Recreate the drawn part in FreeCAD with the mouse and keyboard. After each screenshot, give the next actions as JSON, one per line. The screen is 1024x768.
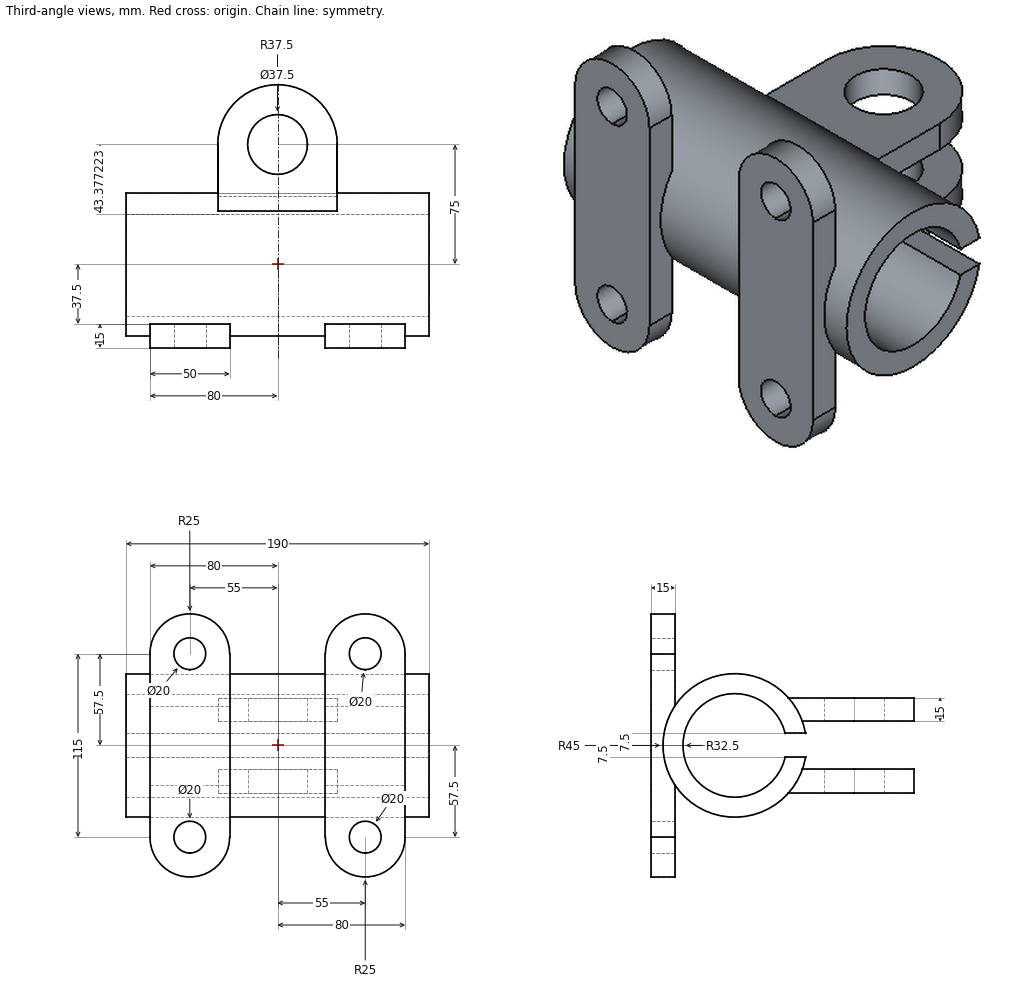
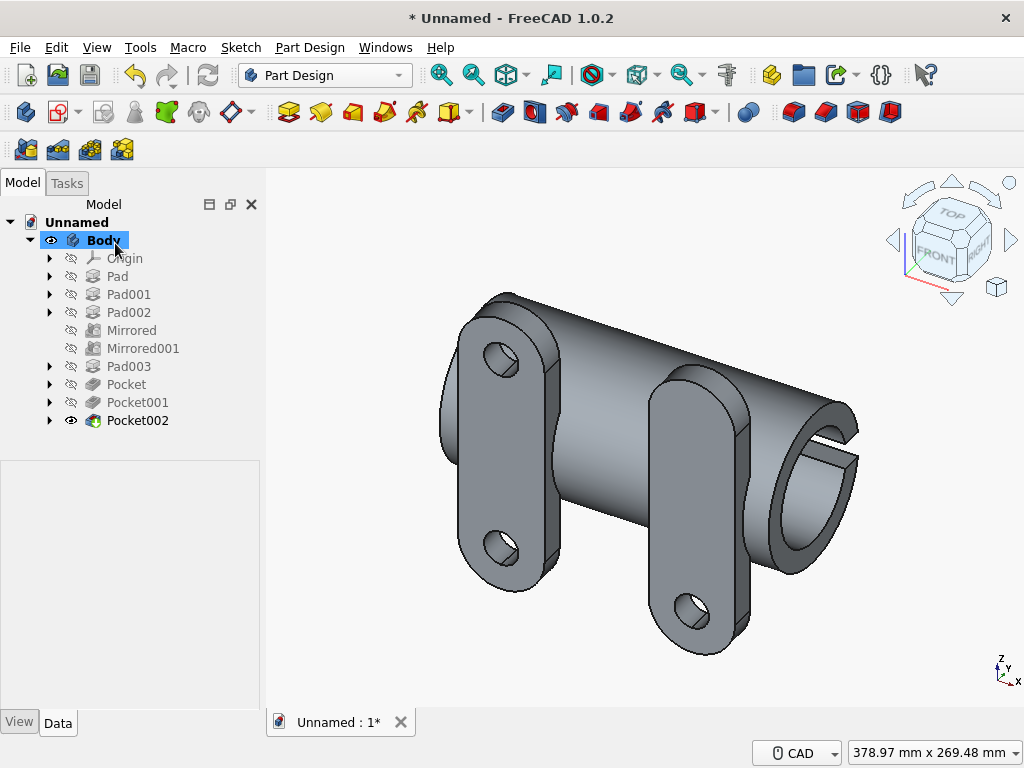
{"action": "left_click", "coordinate": [692, 516]}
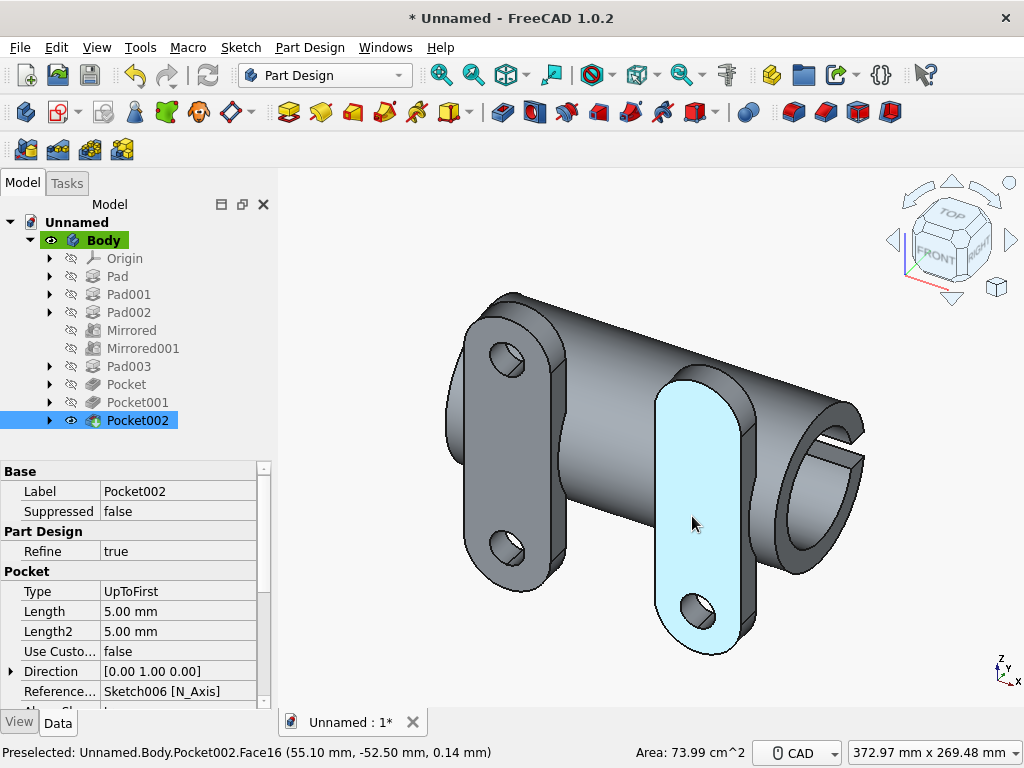
{"action": "left_click", "coordinate": [58, 112]}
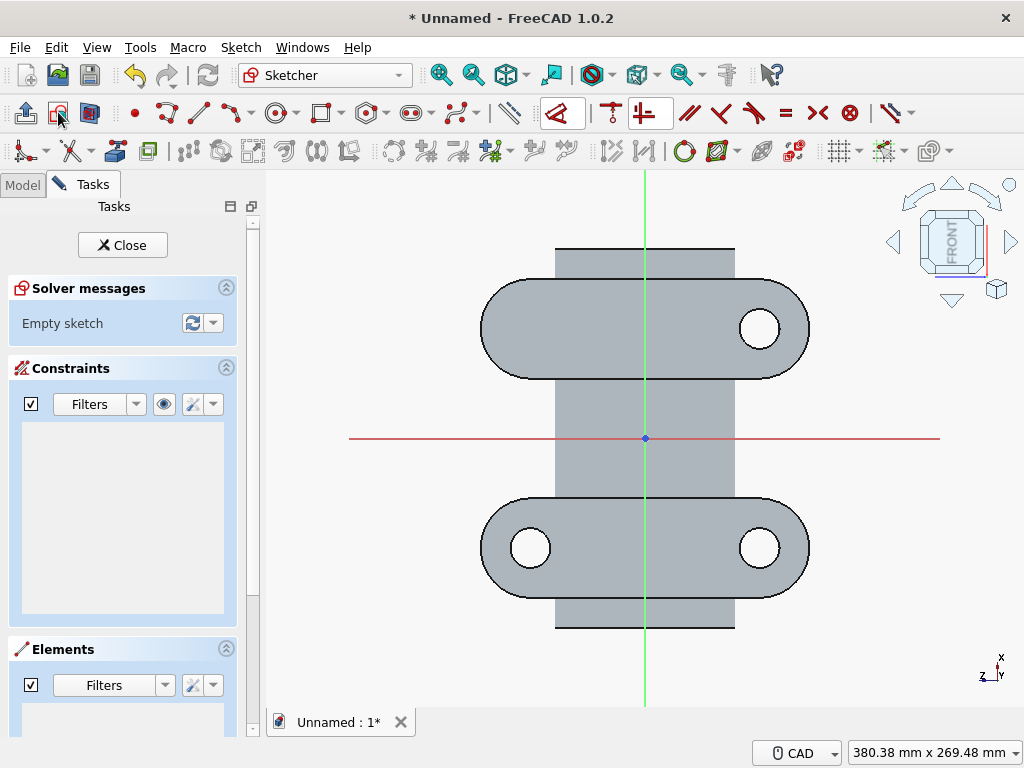
{"action": "scroll", "coordinate": [525, 315], "scroll_direction": "up", "scroll_amount": 11}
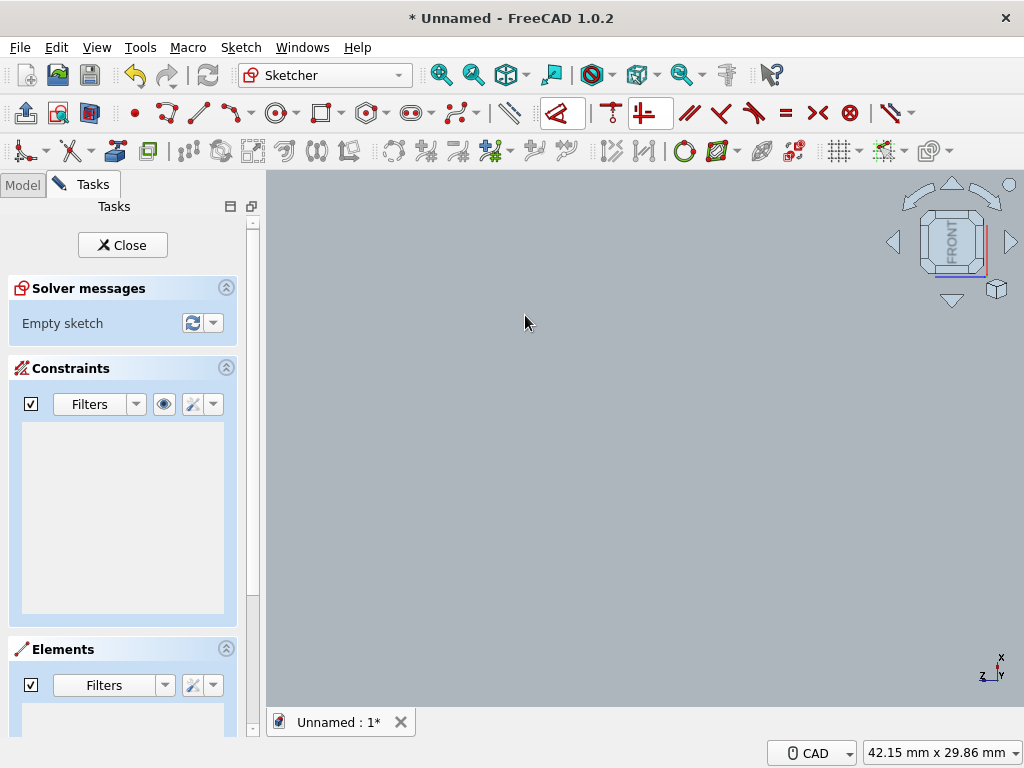
{"action": "left_click", "coordinate": [276, 114]}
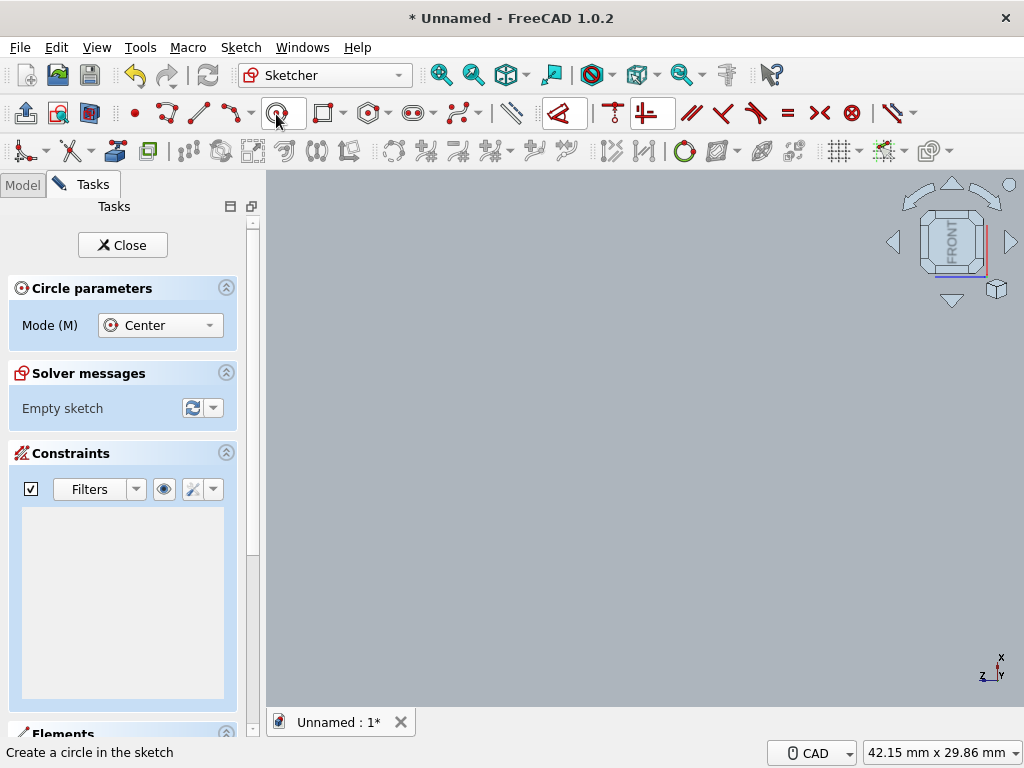
{"action": "left_click", "coordinate": [571, 438]}
{"action": "left_click", "coordinate": [698, 311]}
{"action": "key", "text": "Escape"}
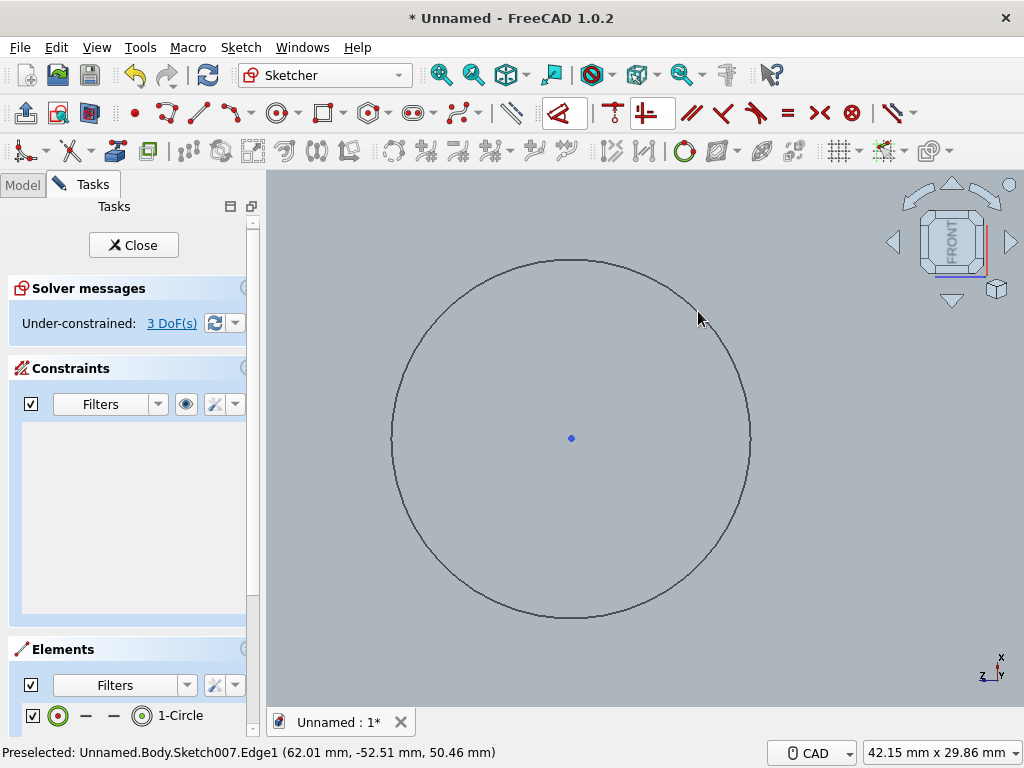
{"action": "left_click", "coordinate": [698, 312]}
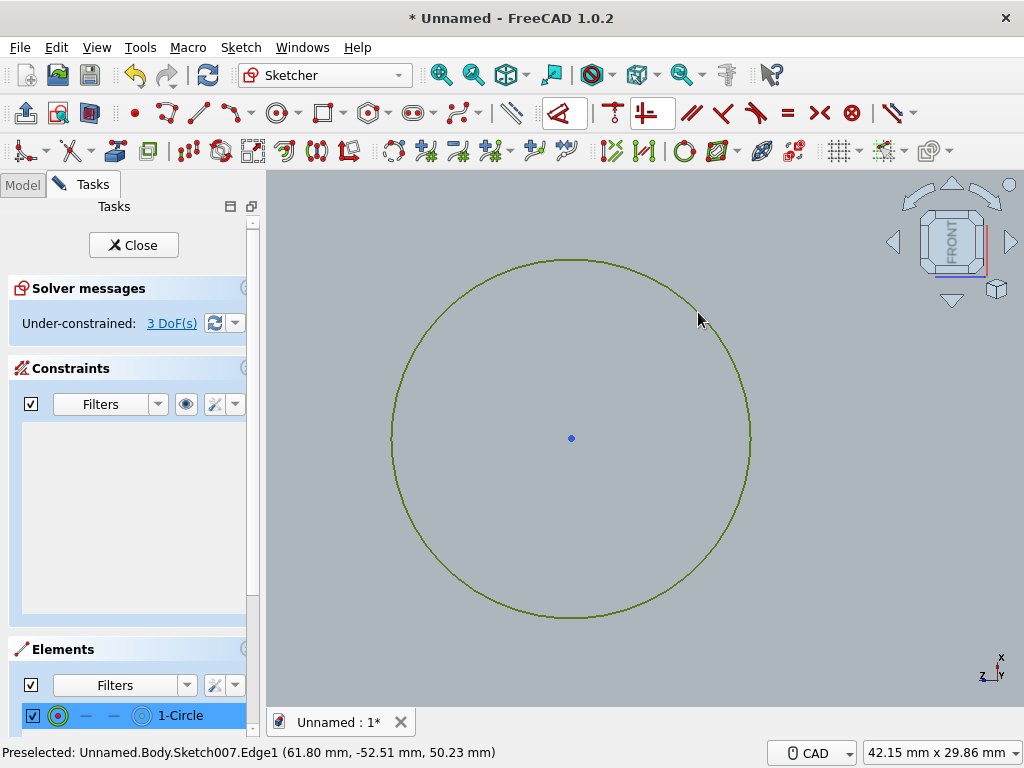
{"action": "left_click", "coordinate": [582, 114]}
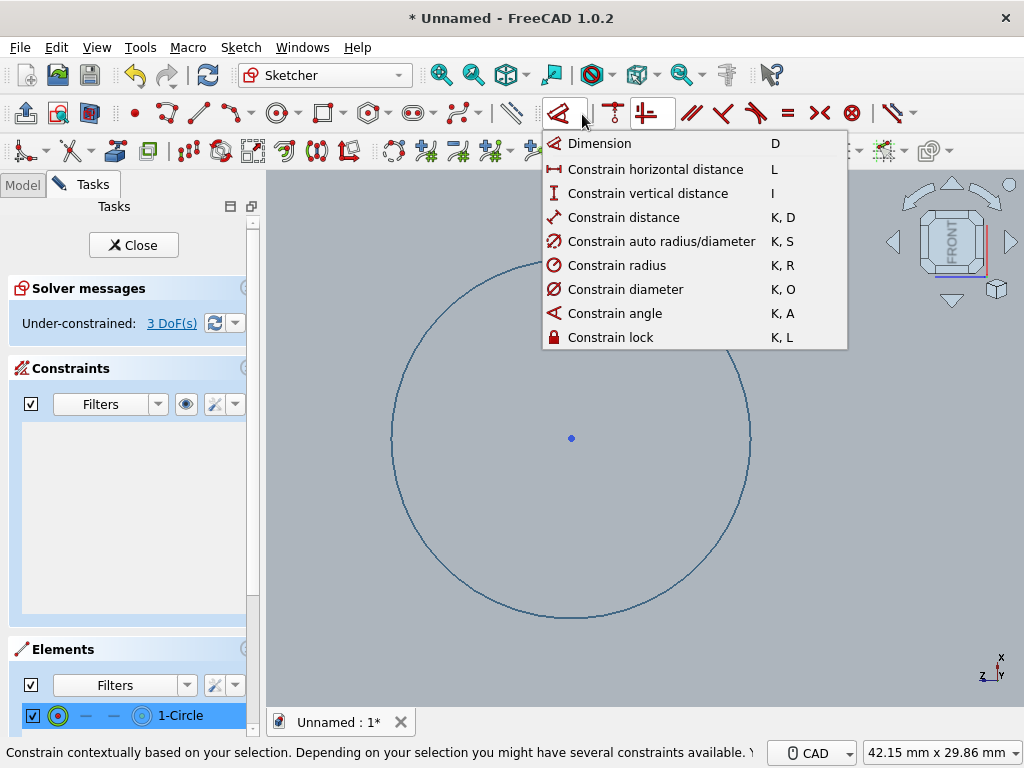
{"action": "left_click", "coordinate": [695, 289]}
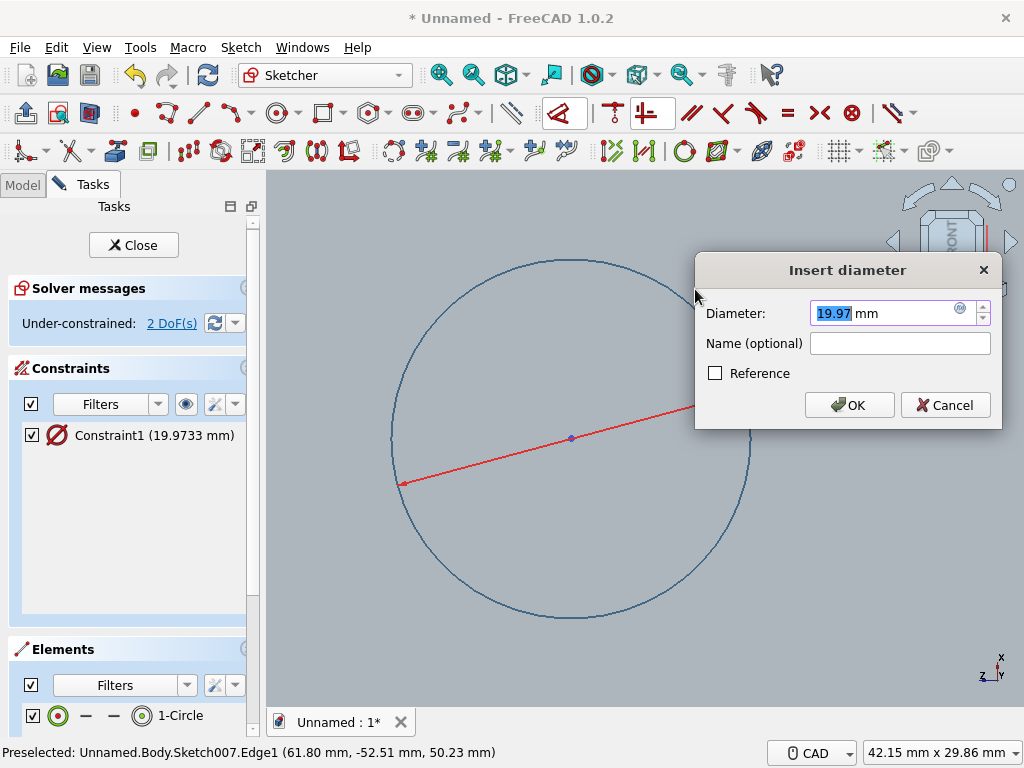
{"action": "type", "text": "20"}
{"action": "key", "text": "Return"}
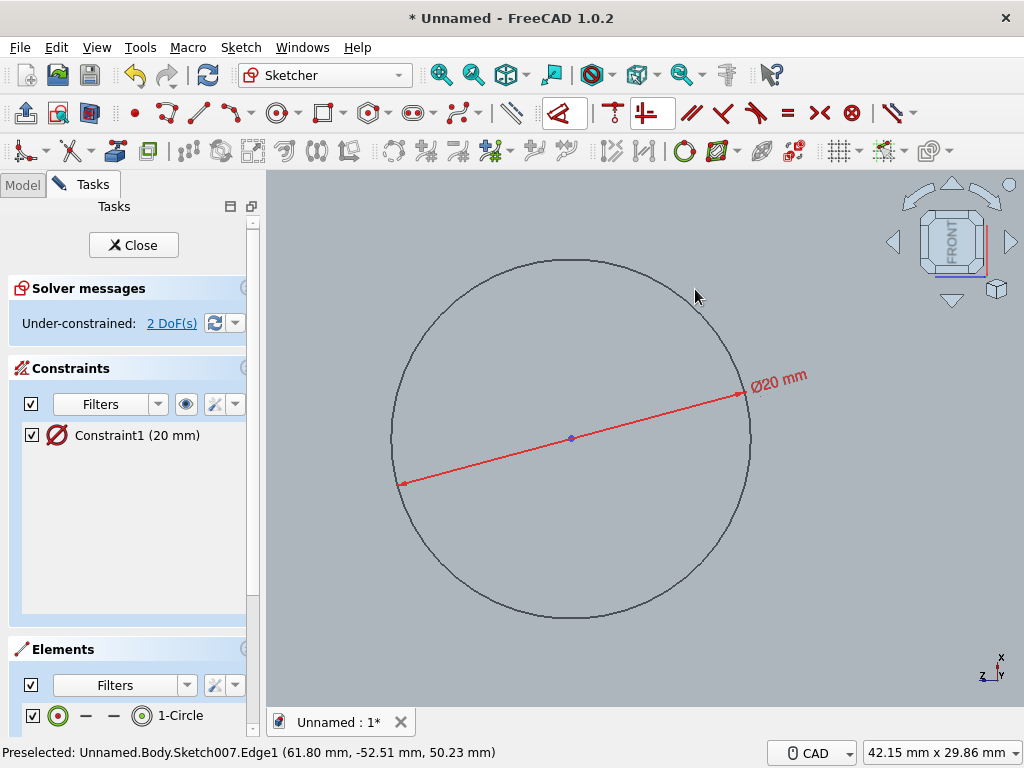
{"action": "left_click", "coordinate": [571, 439]}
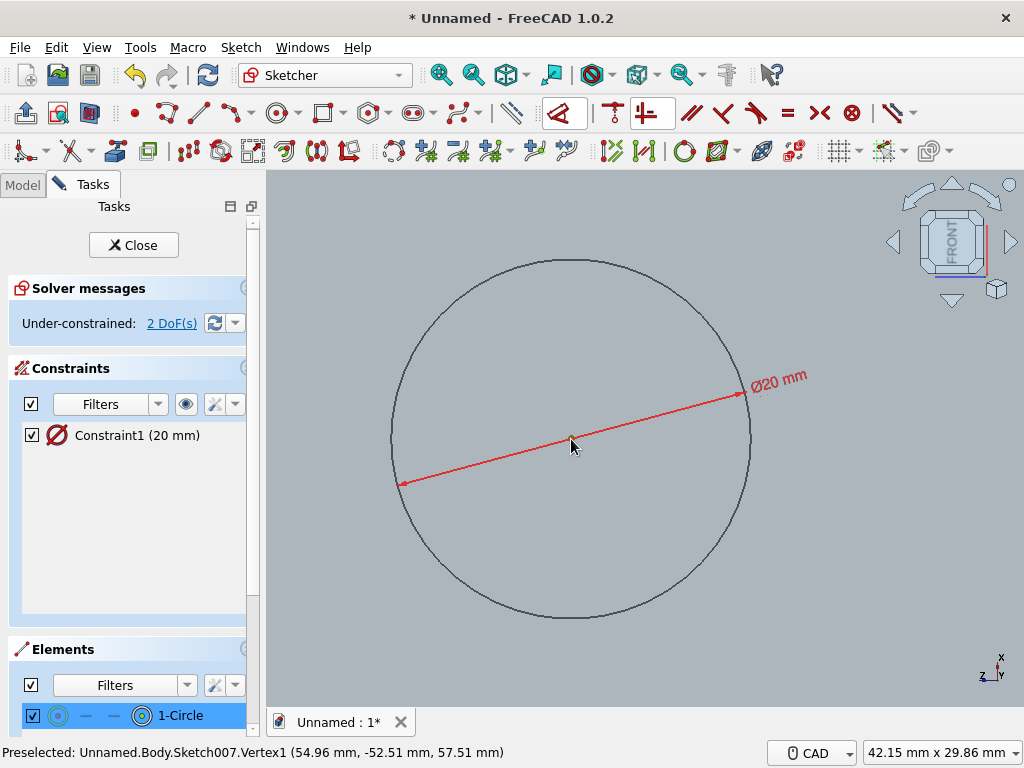
{"action": "left_click", "coordinate": [582, 114]}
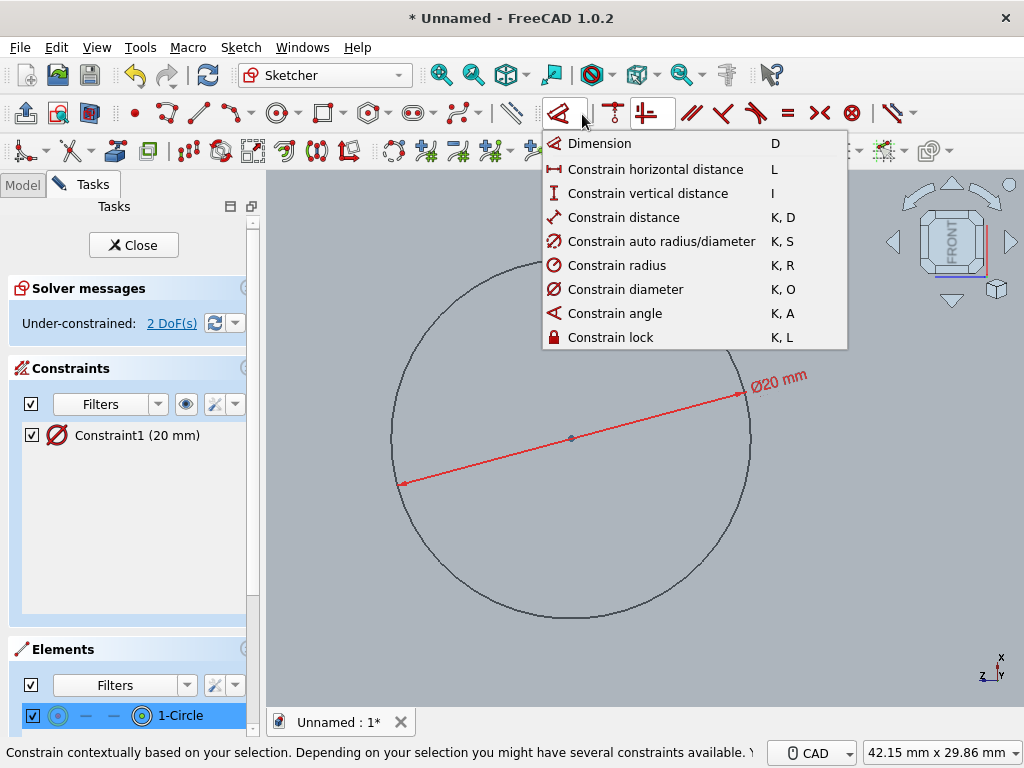
{"action": "left_click", "coordinate": [695, 193]}